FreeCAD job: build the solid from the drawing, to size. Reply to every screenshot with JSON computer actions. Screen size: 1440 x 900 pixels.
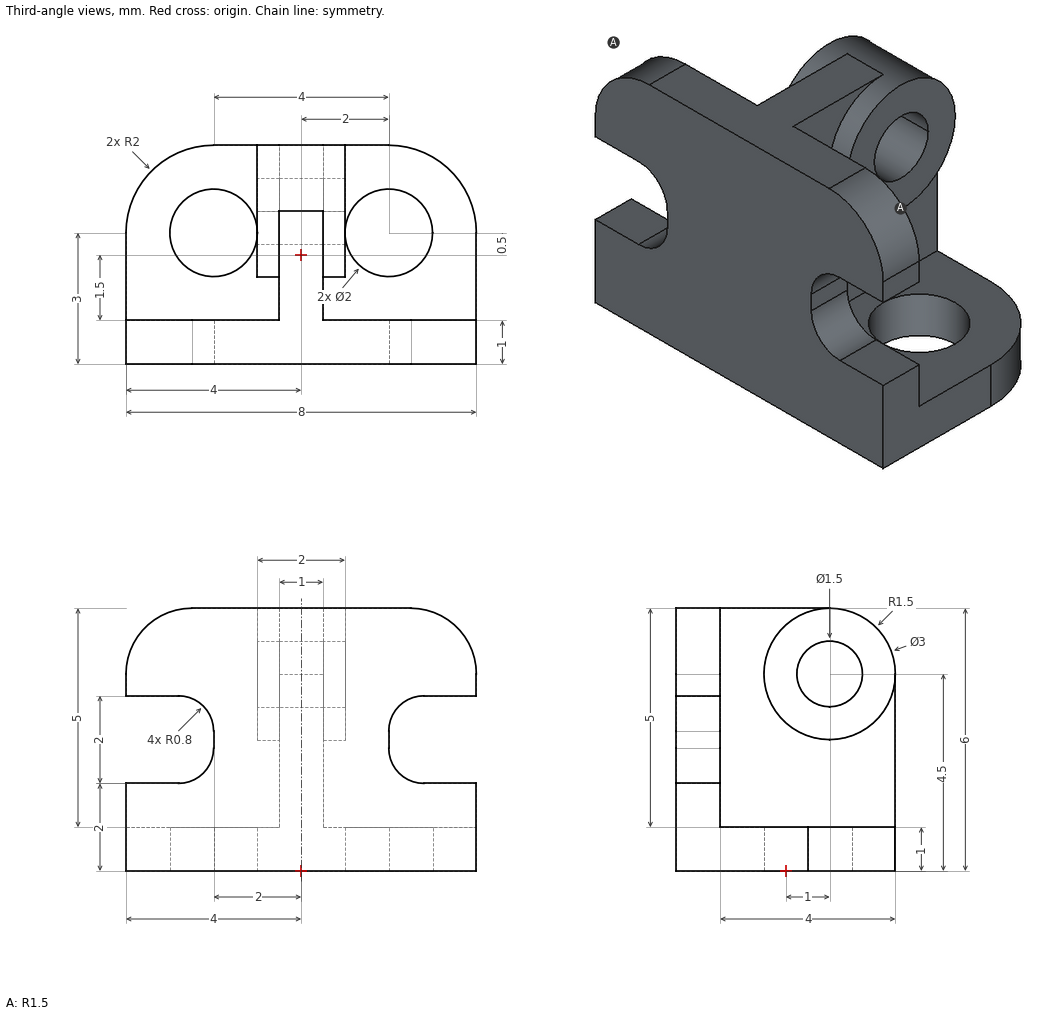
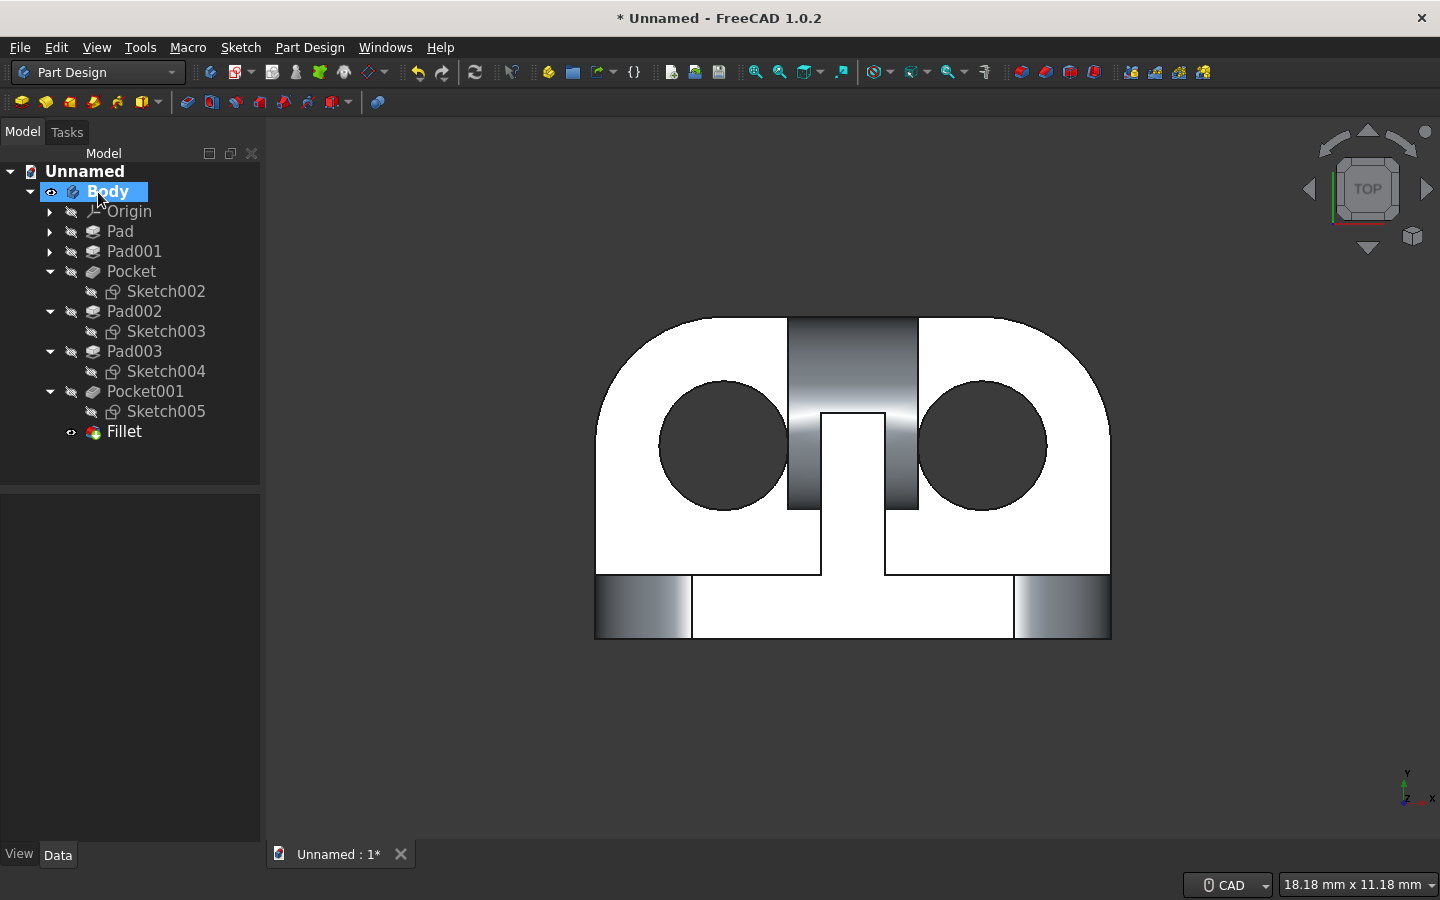
{"action": "key", "text": "0"}